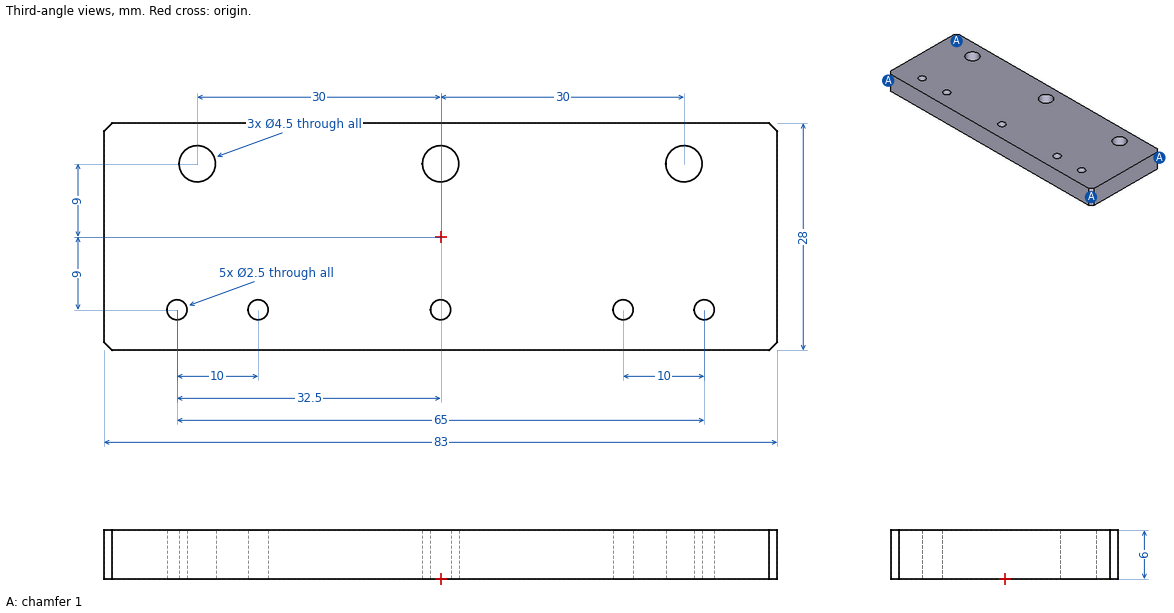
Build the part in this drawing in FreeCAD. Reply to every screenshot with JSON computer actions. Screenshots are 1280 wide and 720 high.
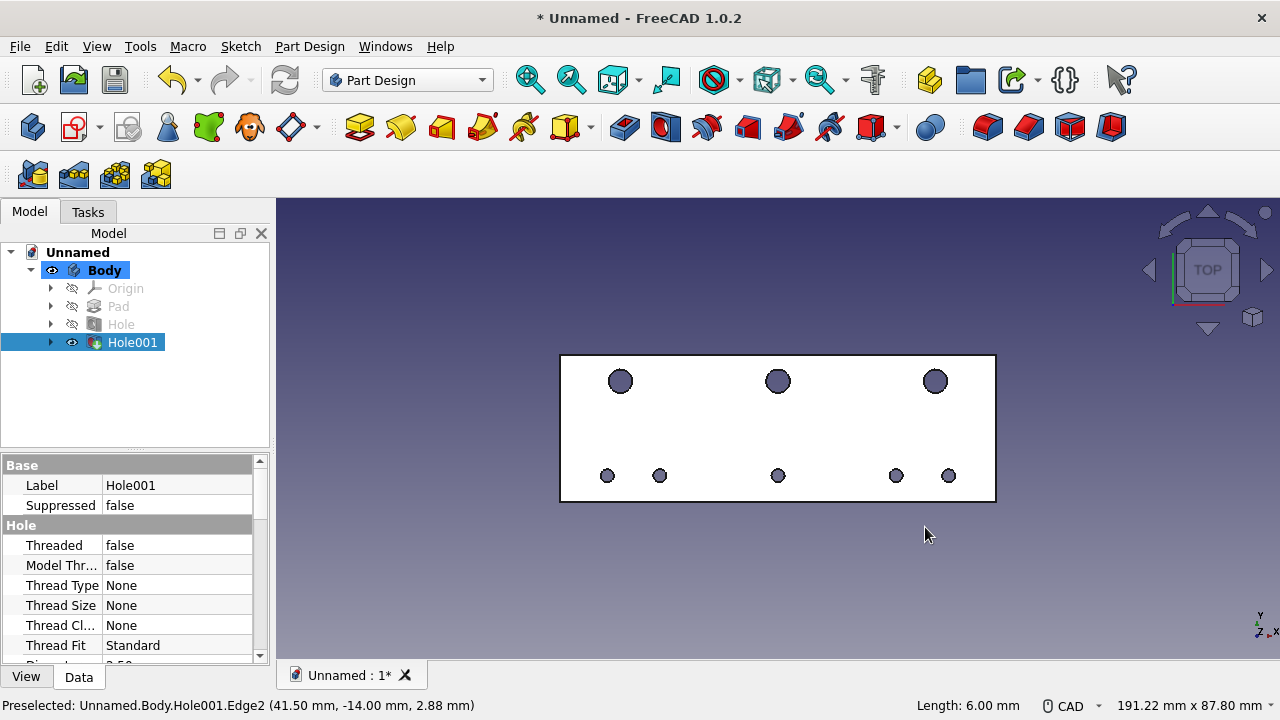
{"action": "key", "text": "1"}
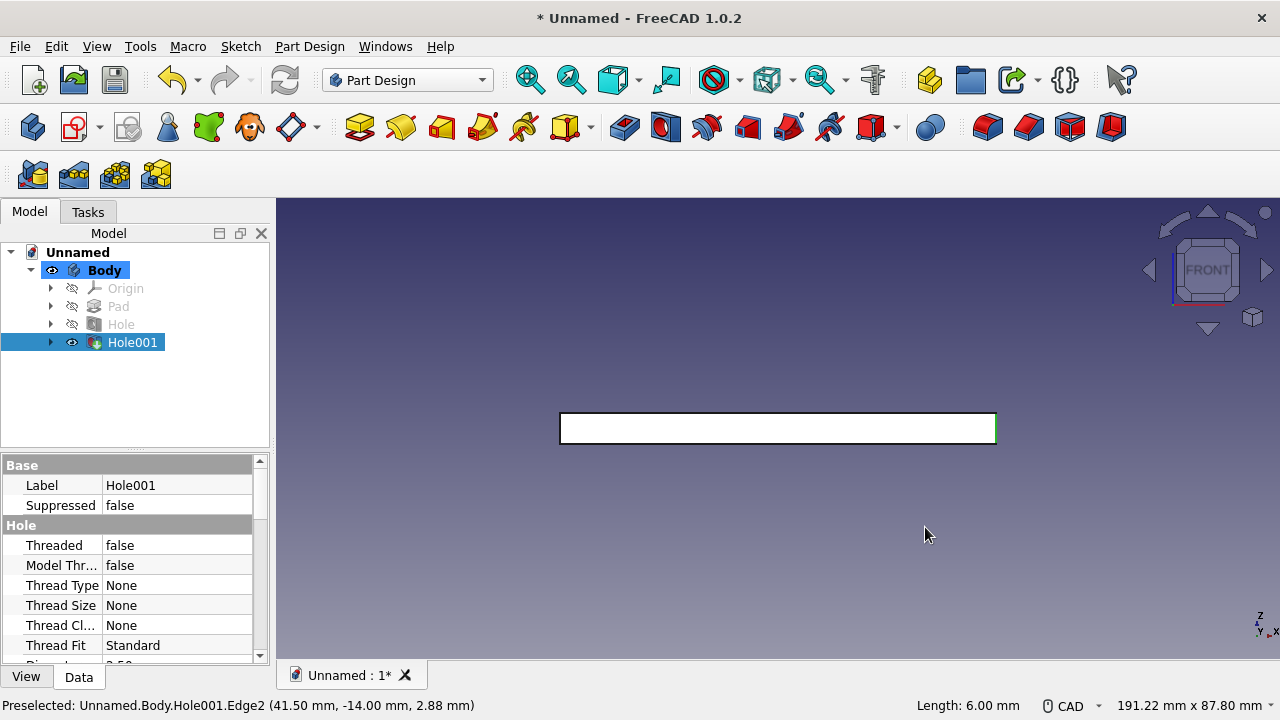
{"action": "left_click", "coordinate": [531, 80]}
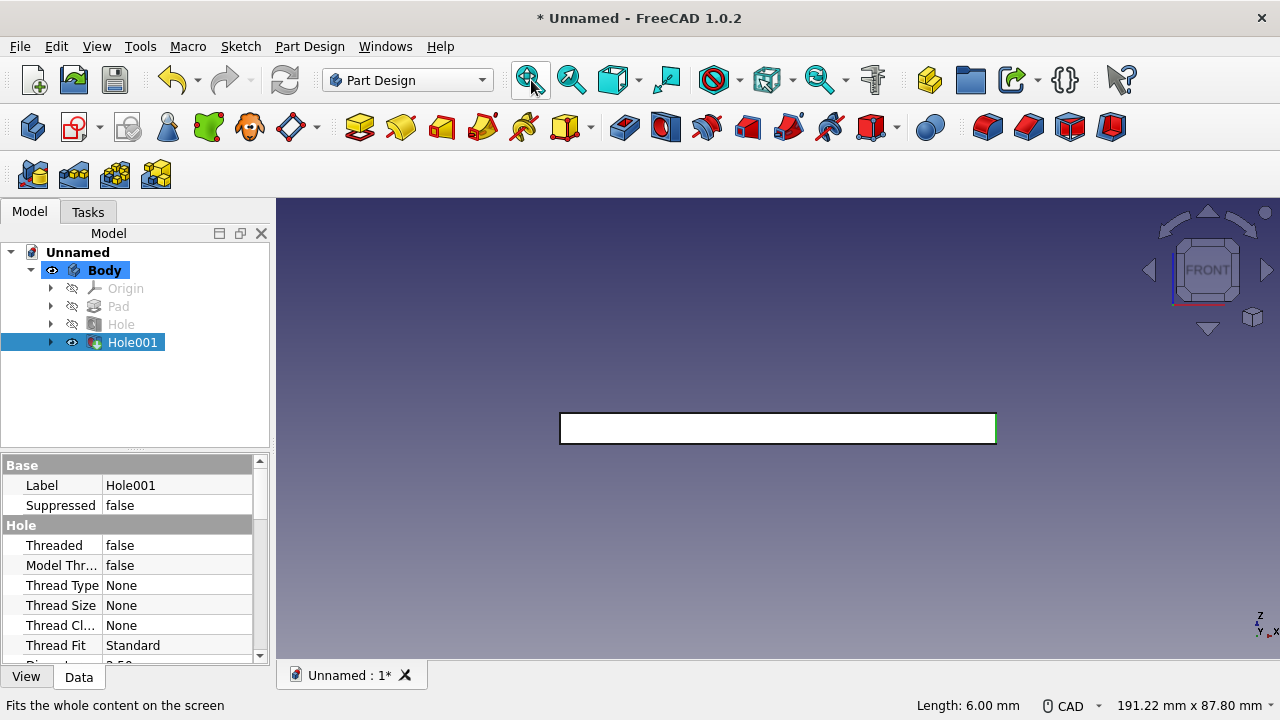
{"action": "left_click", "coordinate": [560, 428], "text": "ctrl"}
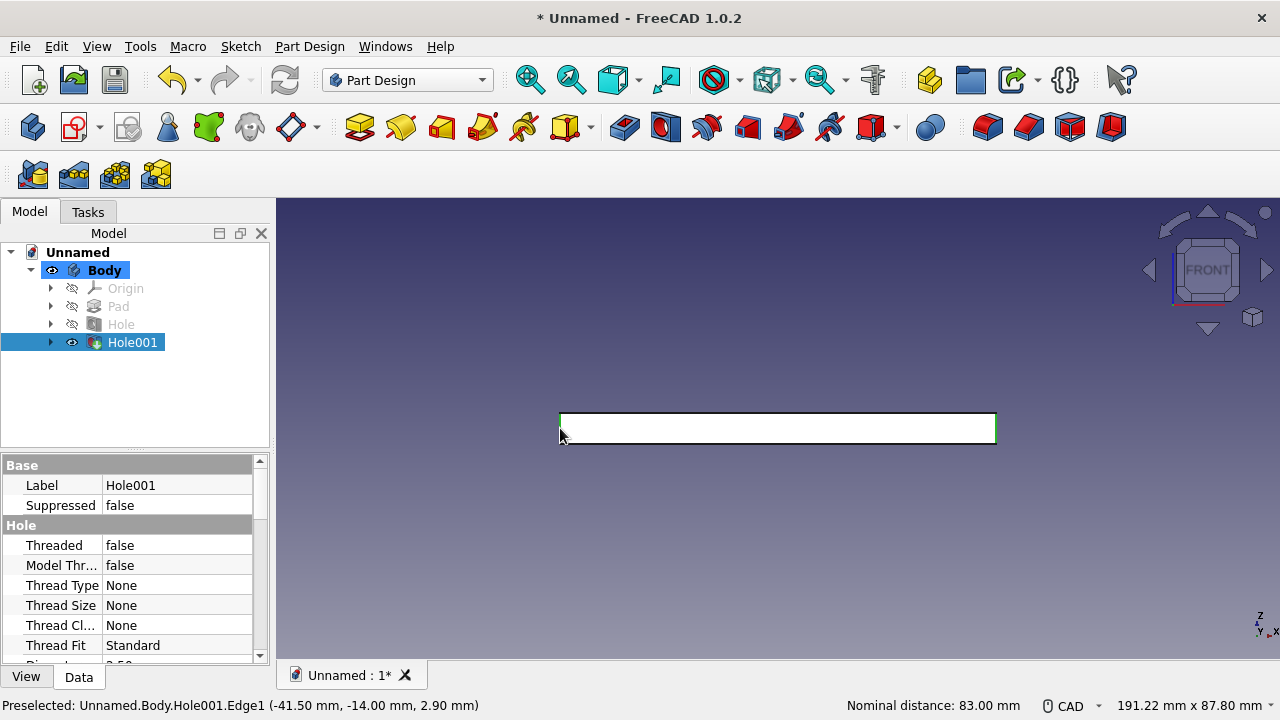
{"action": "key", "text": "3"}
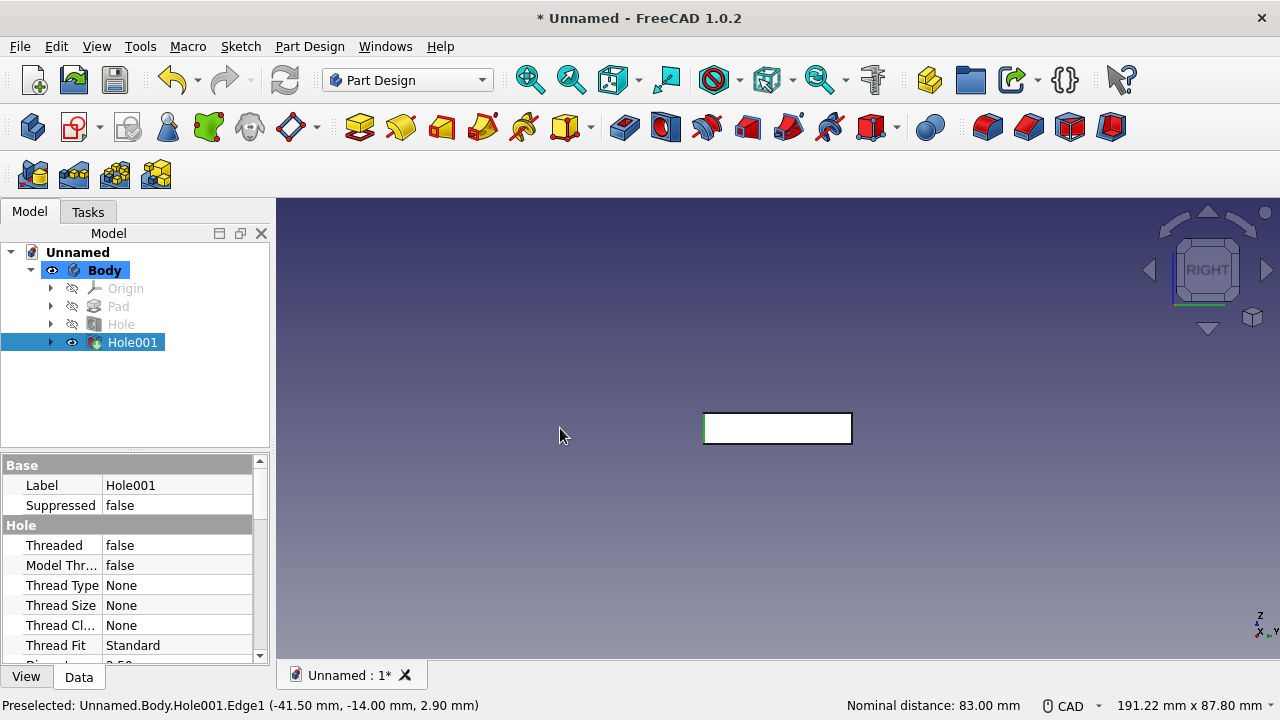
{"action": "left_click", "coordinate": [531, 80]}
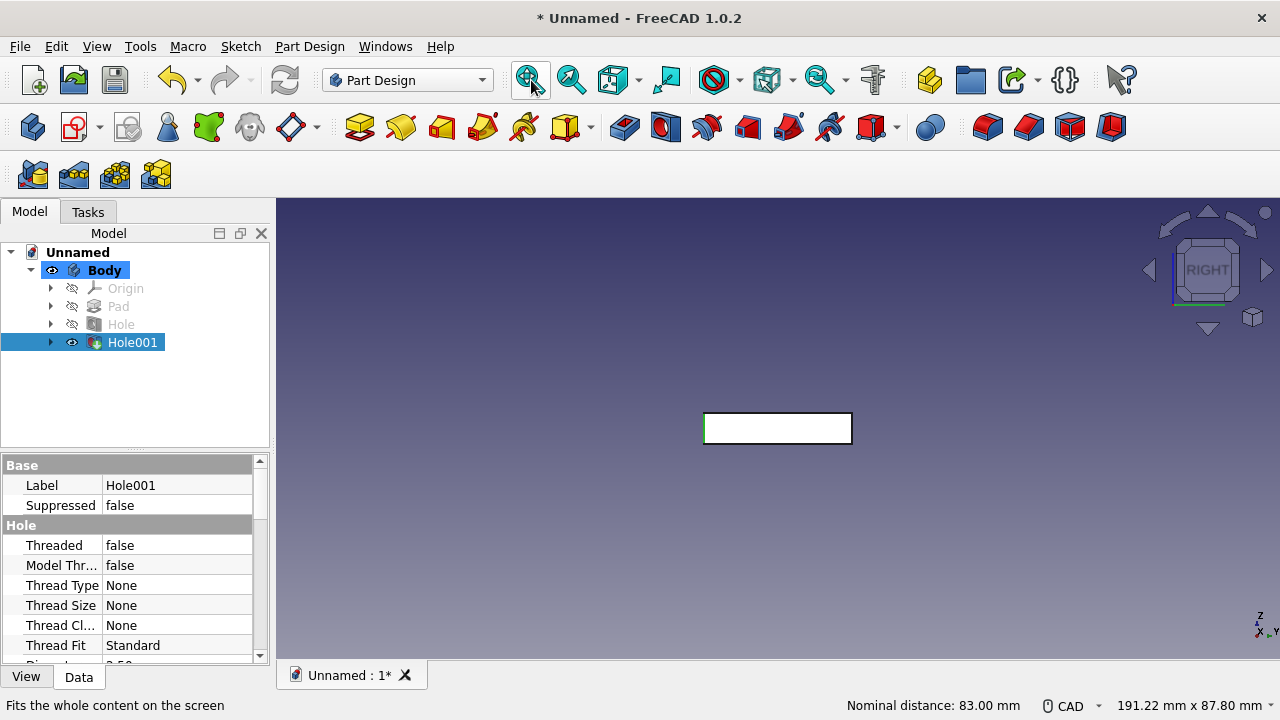
{"action": "left_click", "coordinate": [852, 427], "text": "ctrl"}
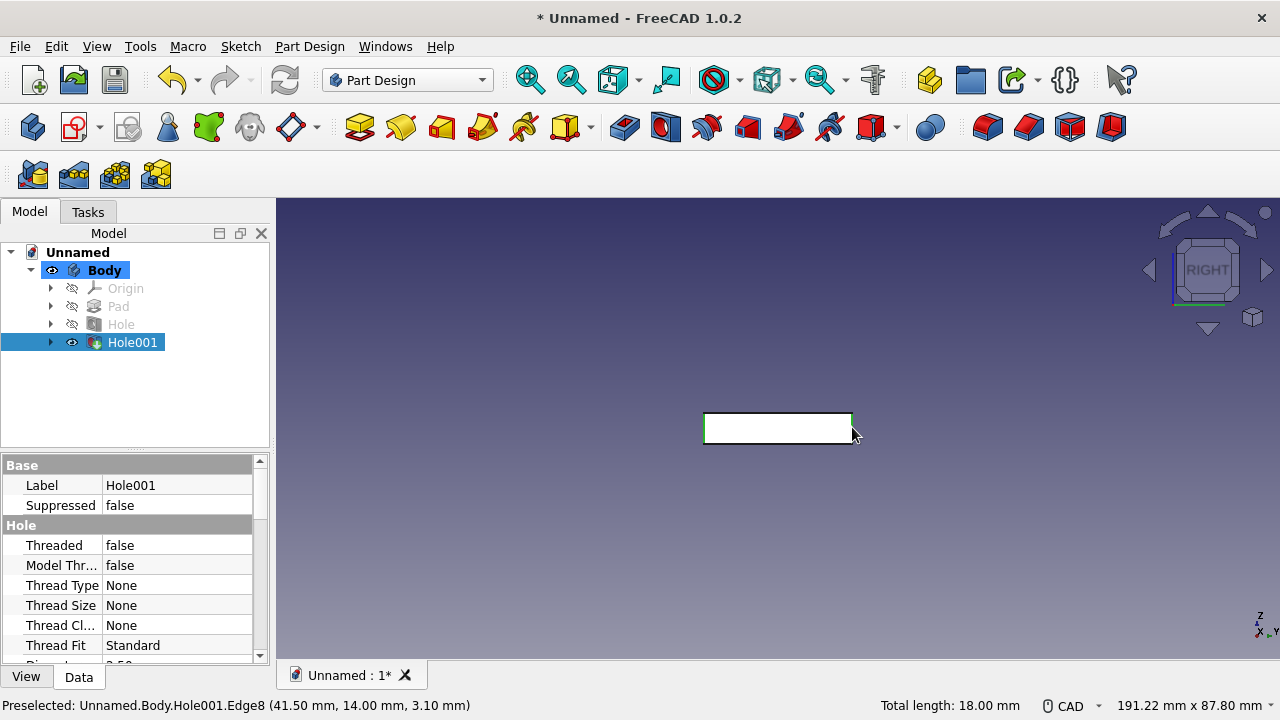
{"action": "key", "text": "5"}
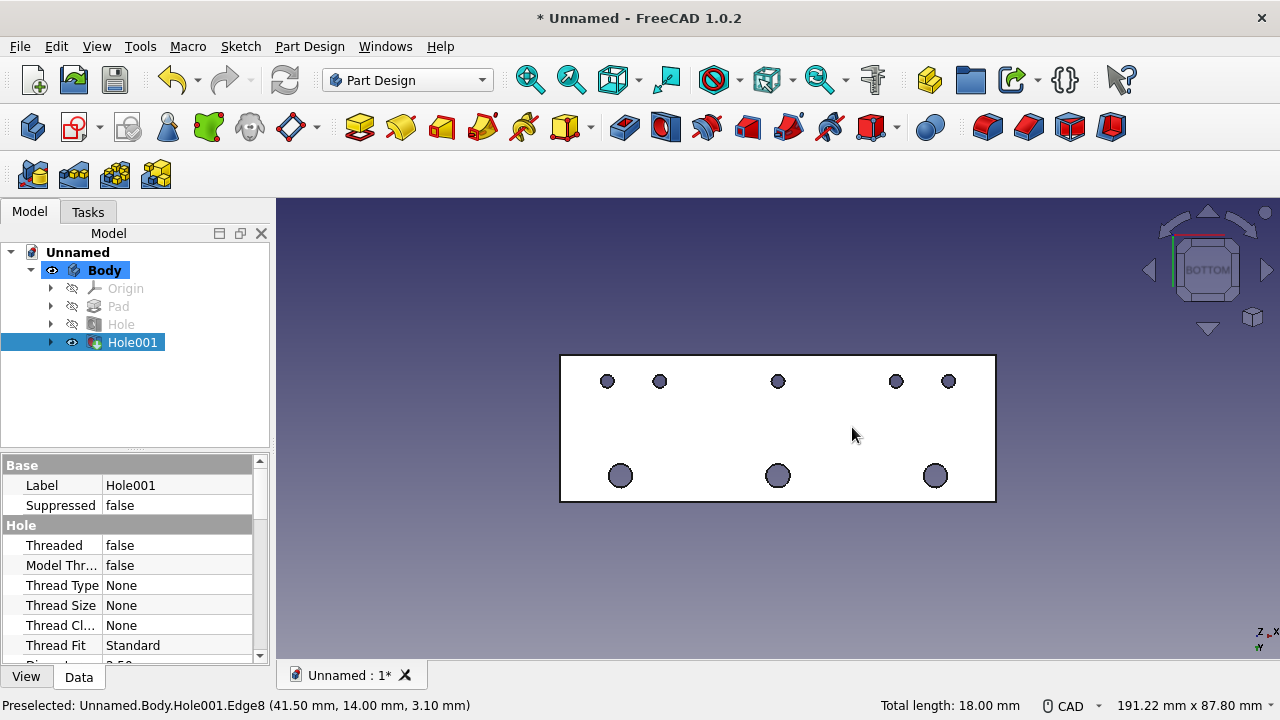
{"action": "left_click", "coordinate": [531, 80]}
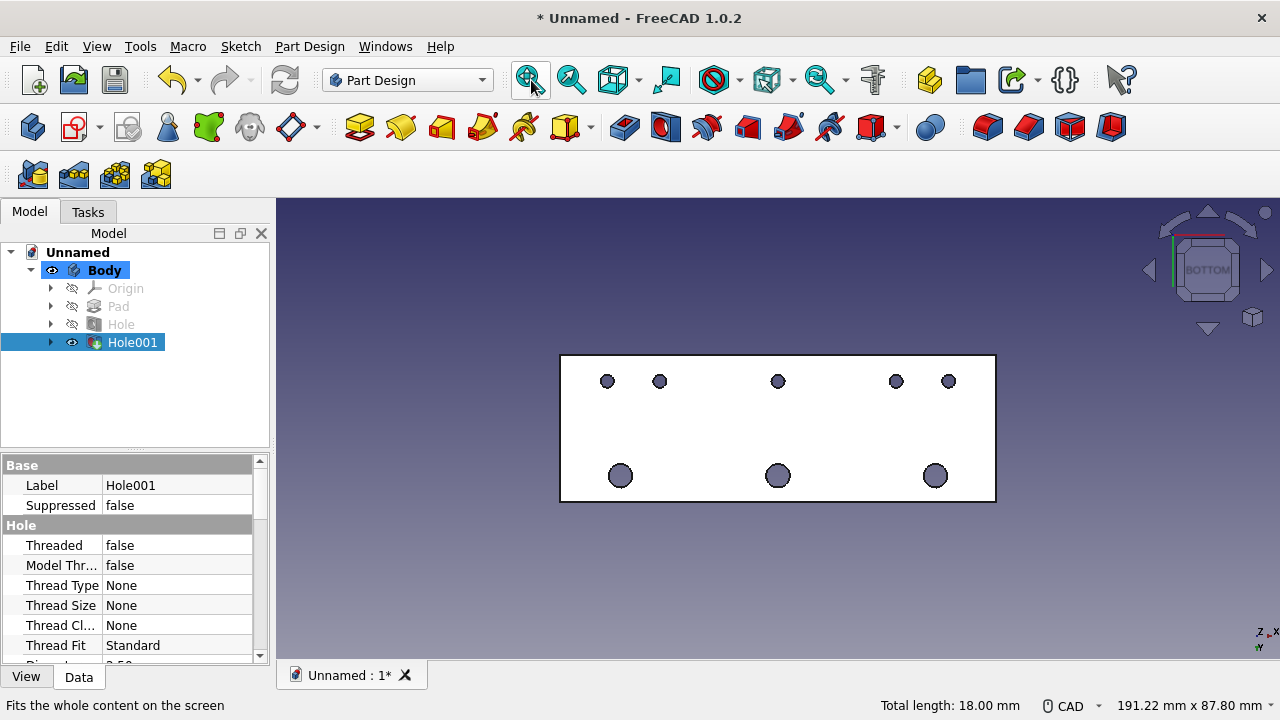
{"action": "key", "text": "4"}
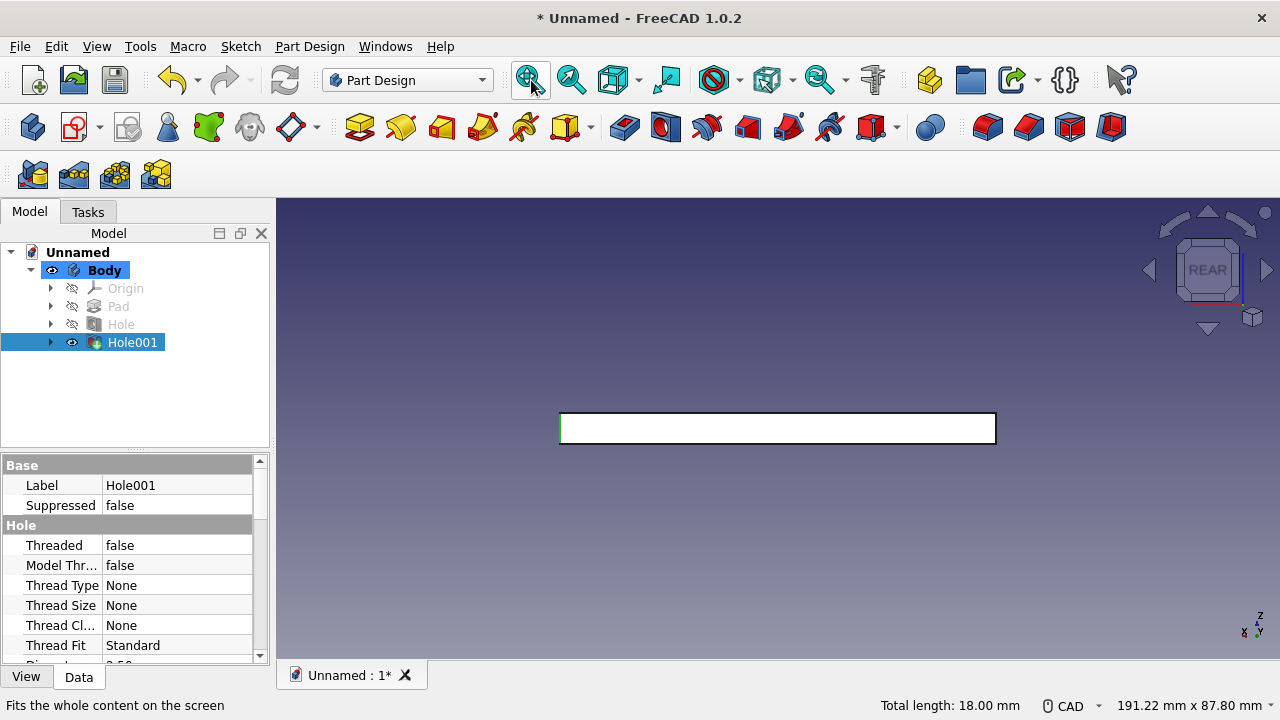
{"action": "key", "text": "v f"}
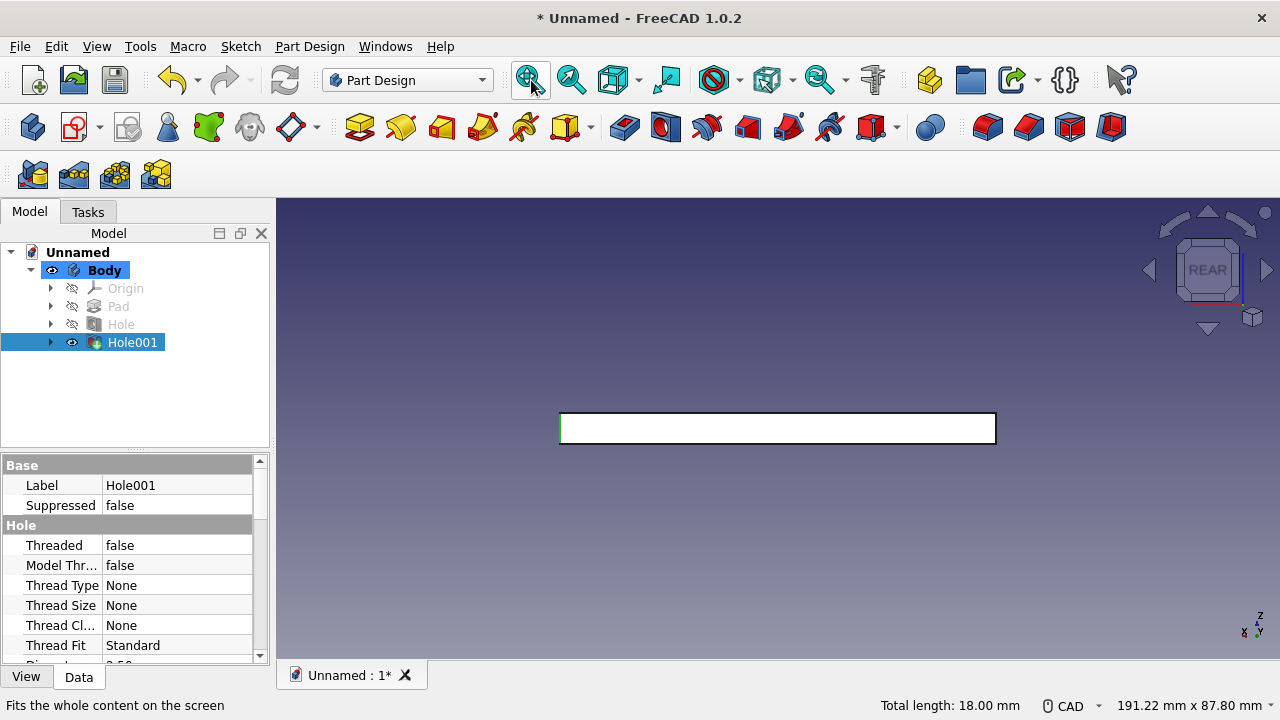
{"action": "left_click", "coordinate": [996, 428], "text": "ctrl"}